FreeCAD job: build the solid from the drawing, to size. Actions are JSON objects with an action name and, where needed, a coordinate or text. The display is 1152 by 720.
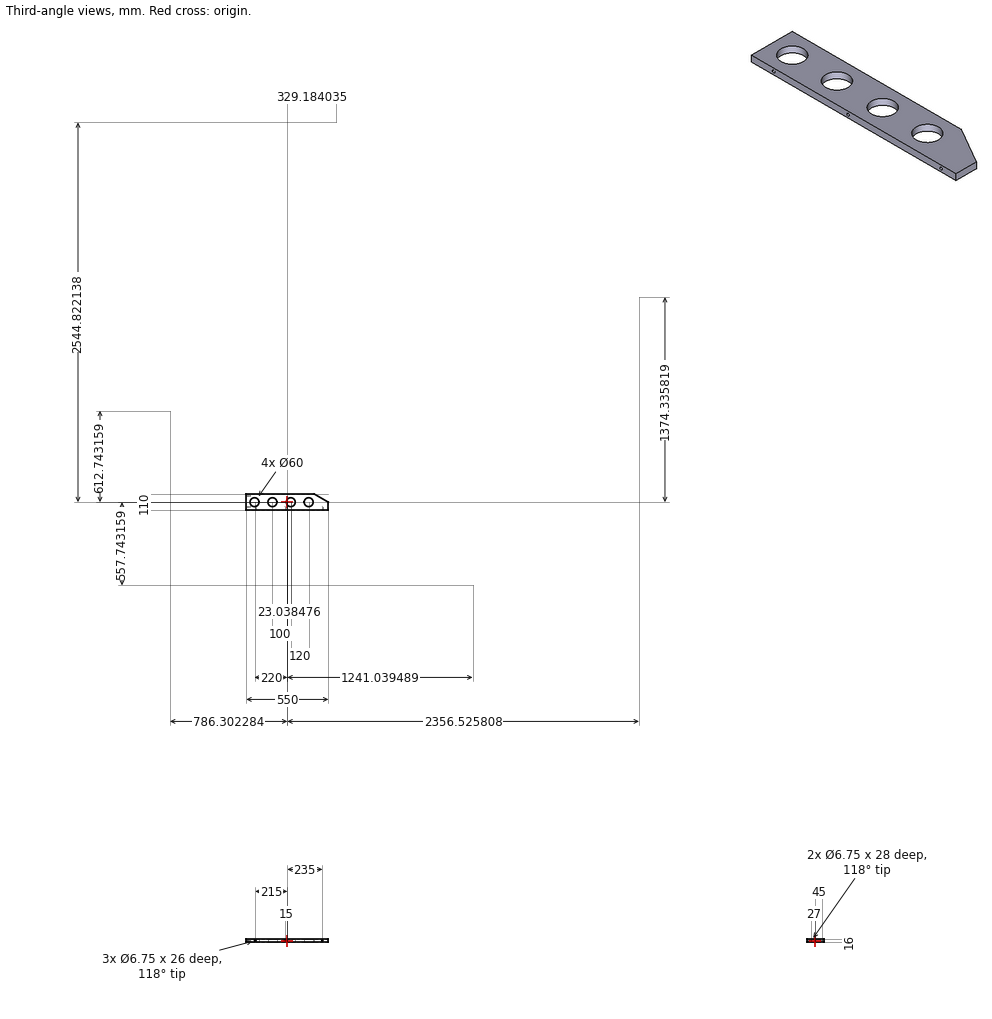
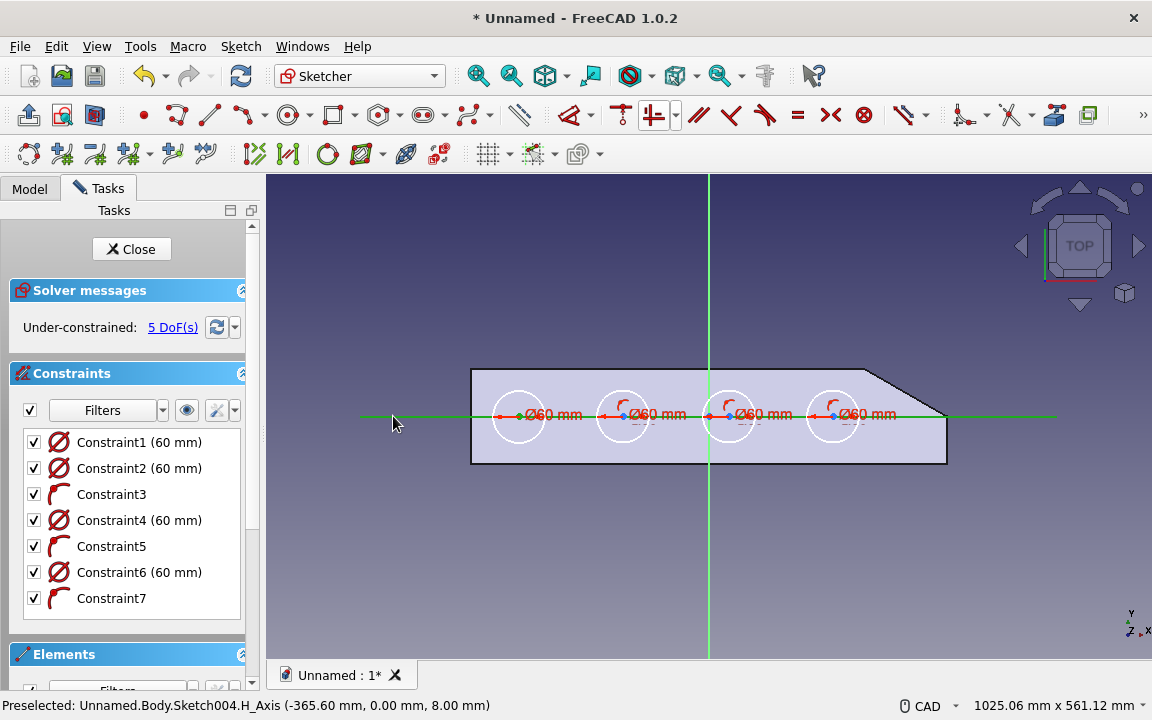
{"action": "key", "text": "c"}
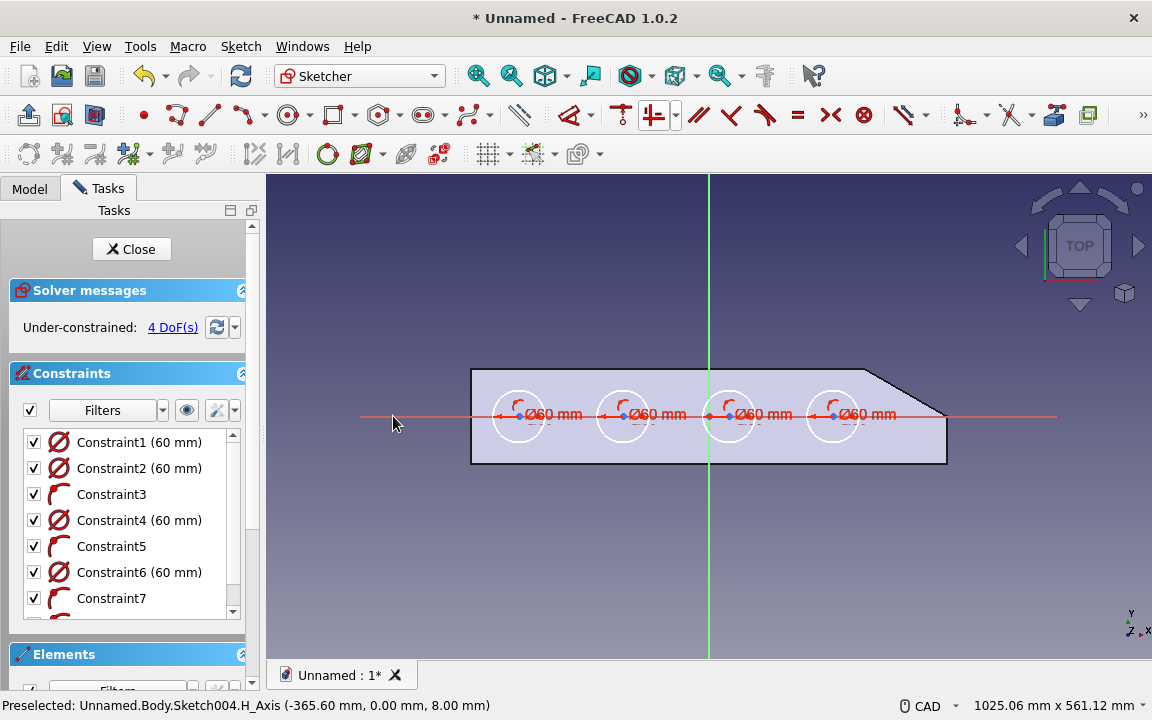
{"action": "key", "text": "d"}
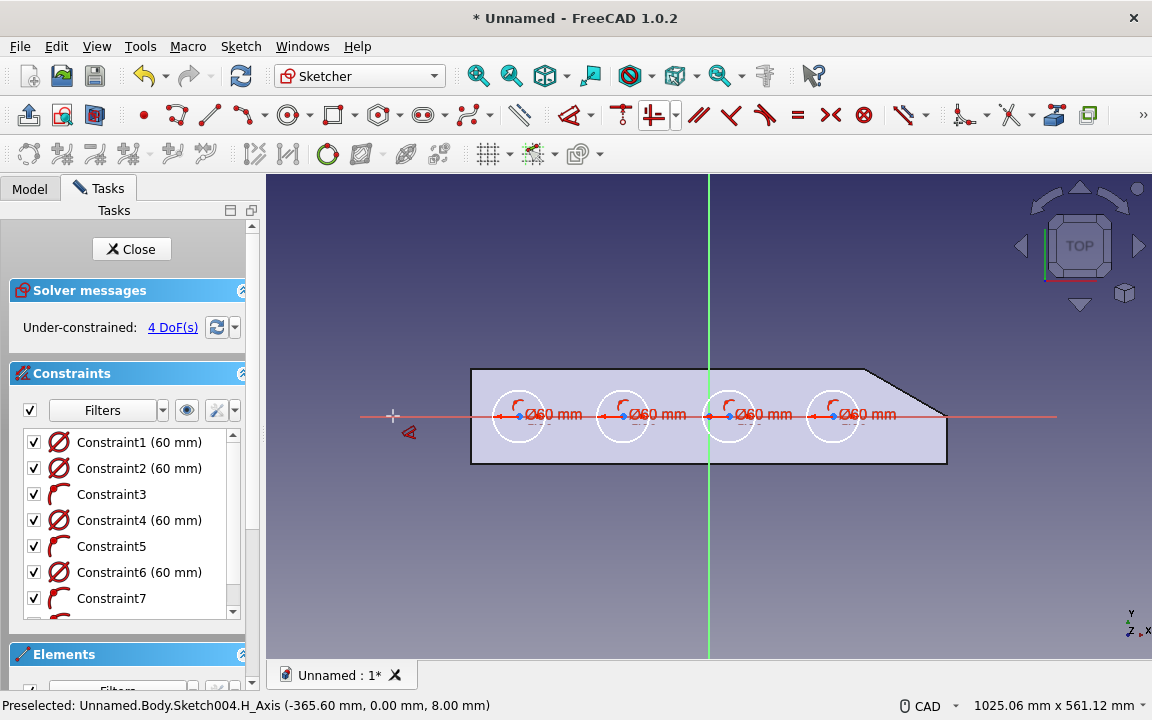
{"action": "left_click", "coordinate": [519, 416]}
{"action": "left_click", "coordinate": [570, 450]}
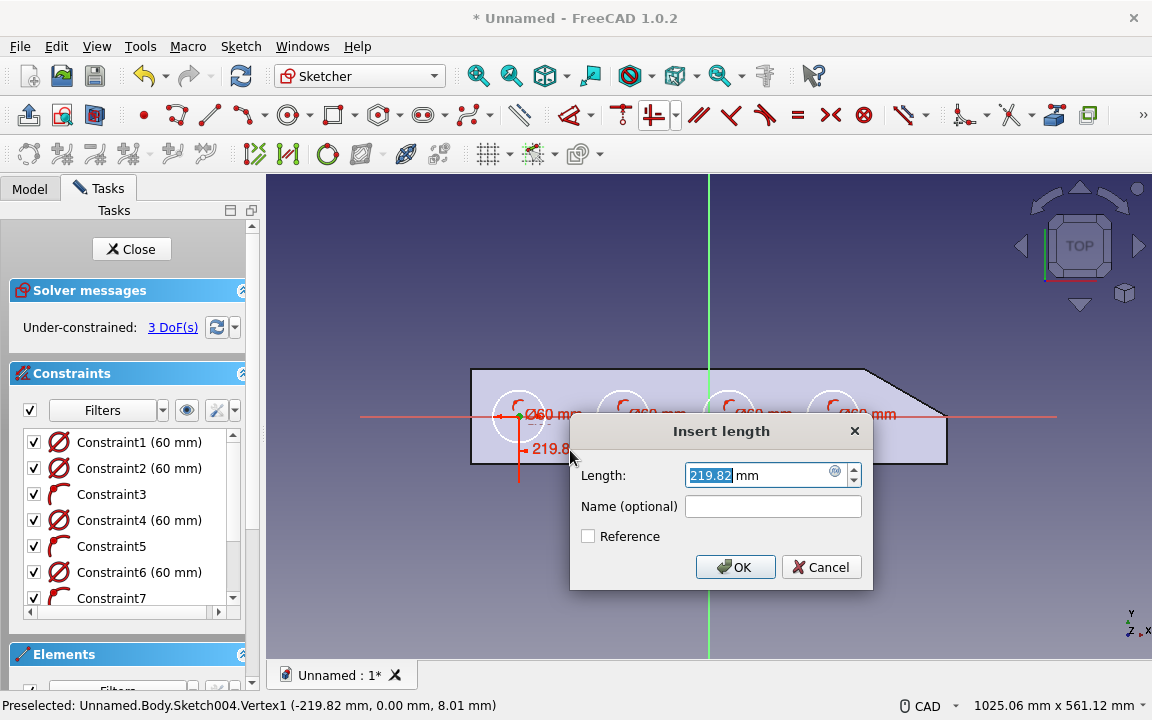
{"action": "type", "text": "220"}
{"action": "key", "text": "Return"}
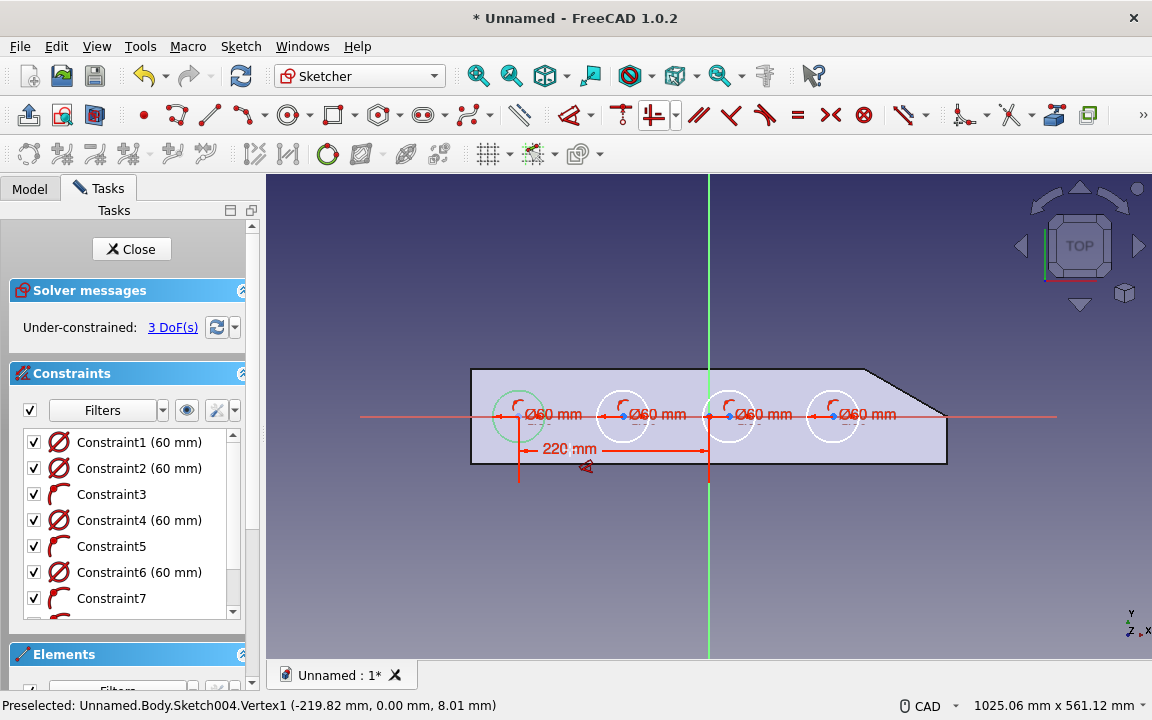
{"action": "left_click", "coordinate": [623, 416]}
{"action": "left_click", "coordinate": [666, 450]}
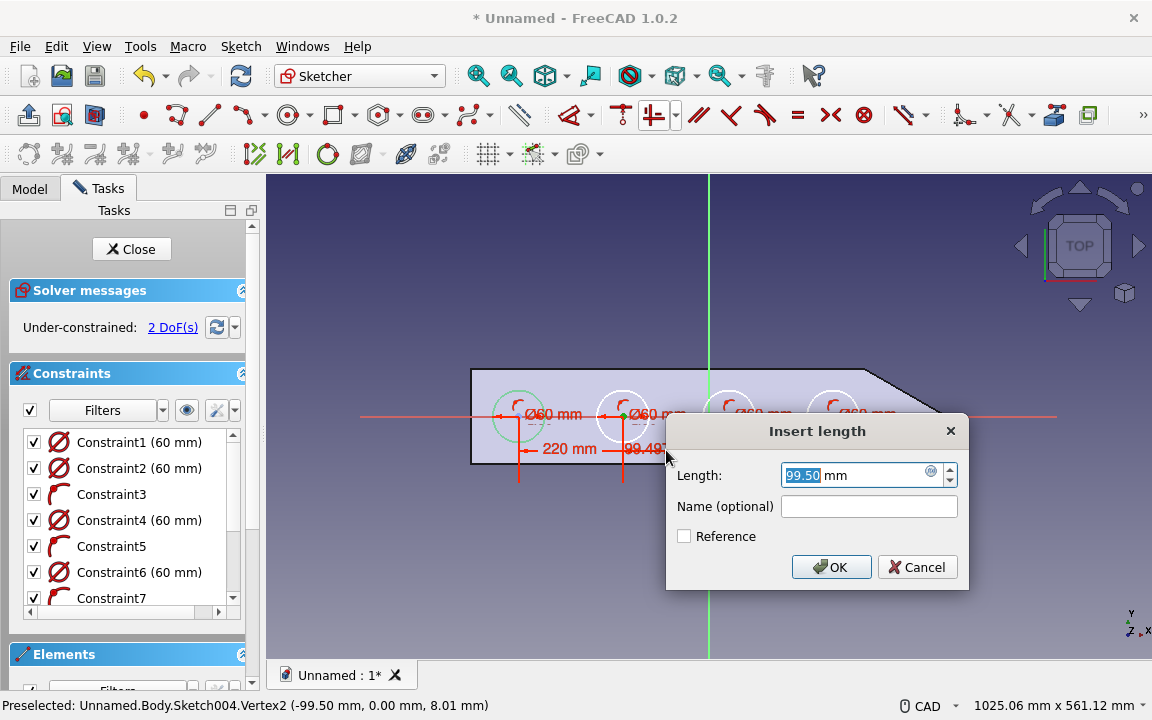
{"action": "type", "text": "100"}
{"action": "key", "text": "Return"}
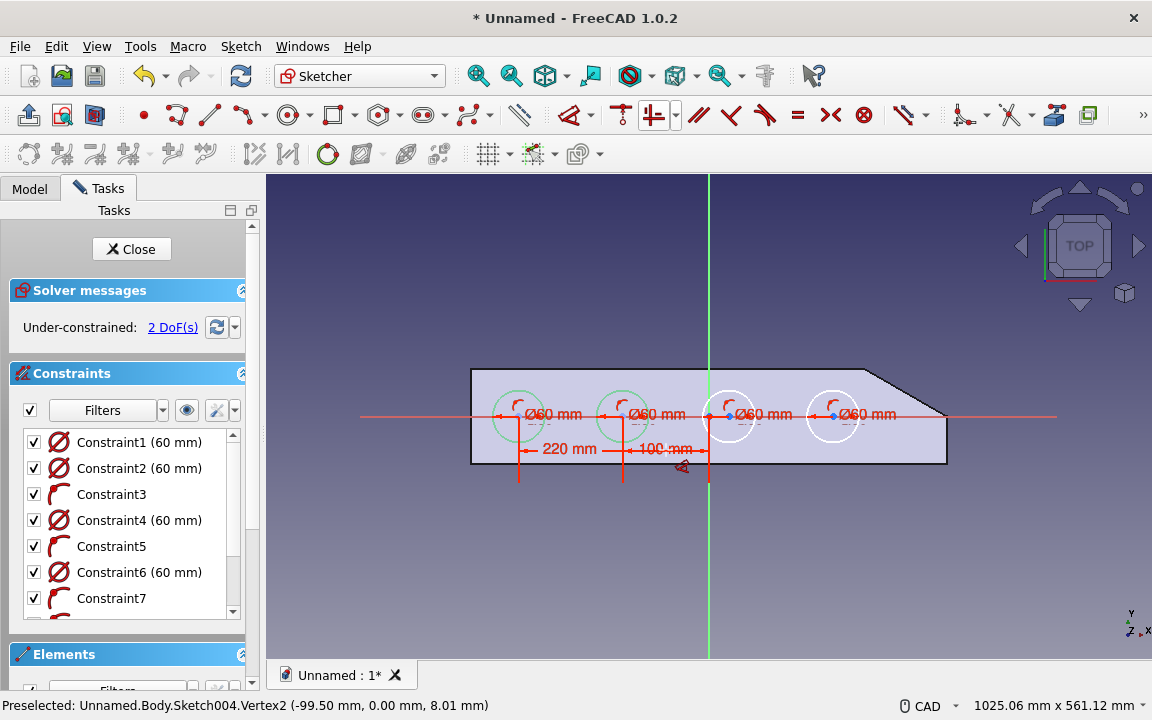
{"action": "left_click", "coordinate": [729, 416]}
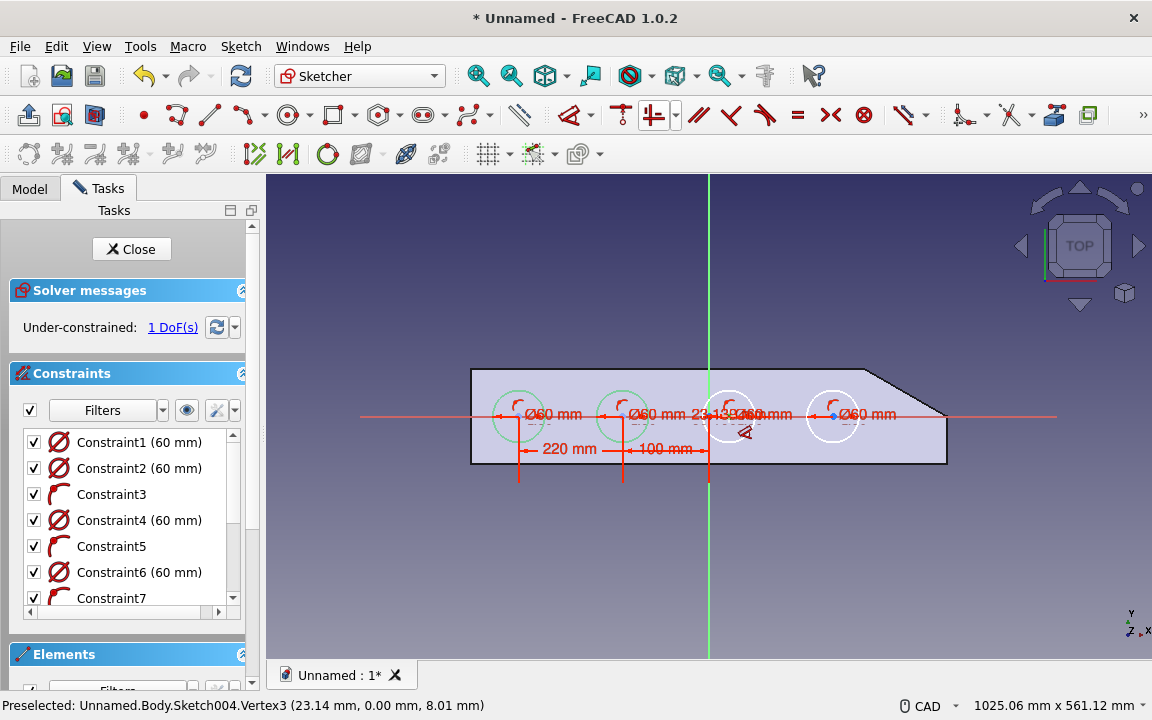
{"action": "left_click", "coordinate": [833, 416]}
{"action": "left_click", "coordinate": [781, 450]}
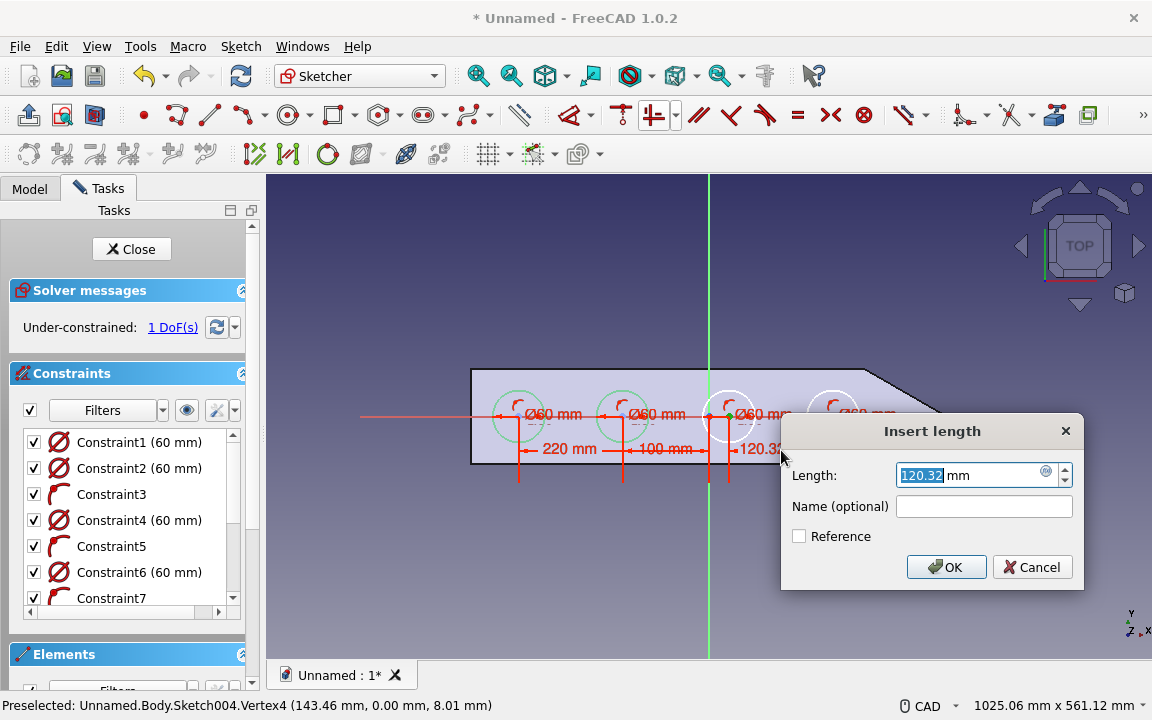
{"action": "type", "text": "120"}
{"action": "key", "text": "Return"}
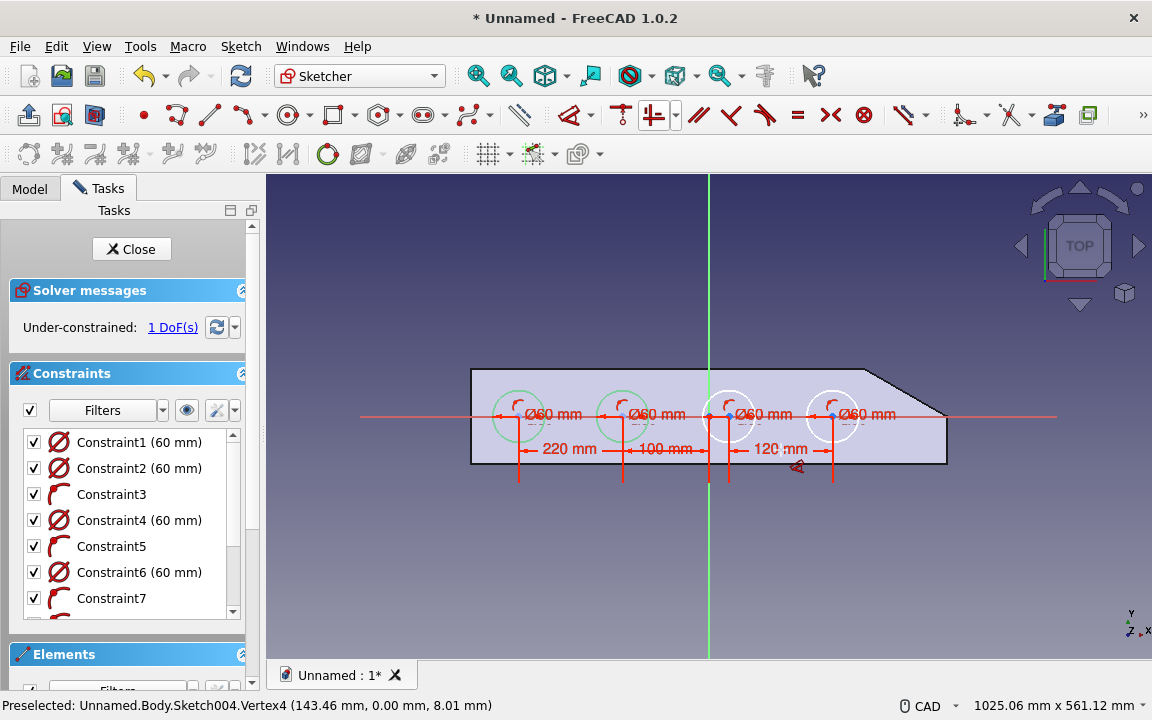
{"action": "scroll", "coordinate": [729, 416], "scroll_direction": "up", "scroll_amount": 4}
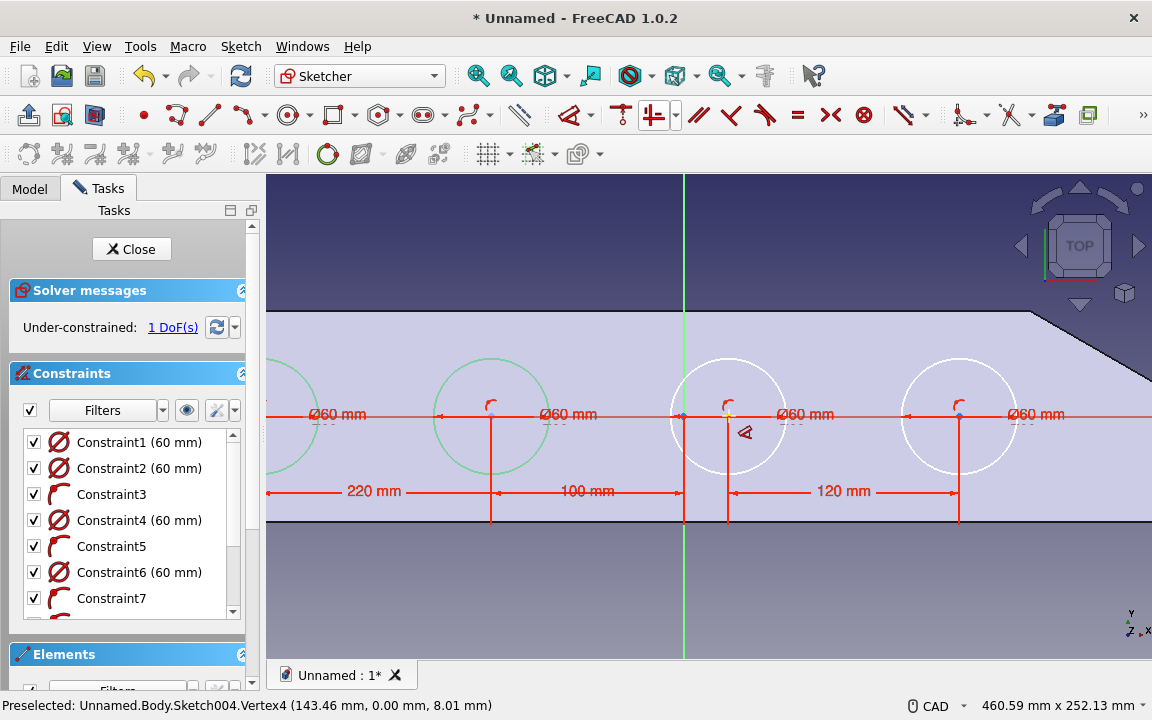
{"action": "left_click", "coordinate": [728, 416]}
{"action": "left_click", "coordinate": [706, 450]}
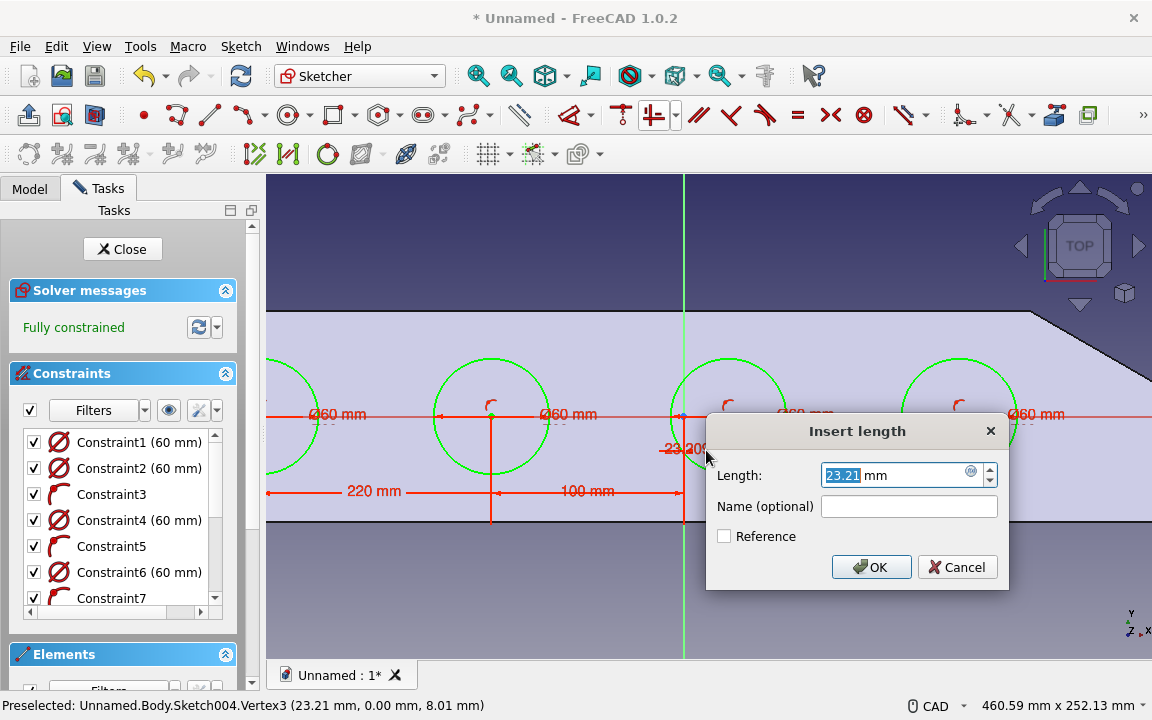
{"action": "type", "text": "23.038476"}
{"action": "key", "text": "Return"}
{"action": "key", "text": "Escape"}